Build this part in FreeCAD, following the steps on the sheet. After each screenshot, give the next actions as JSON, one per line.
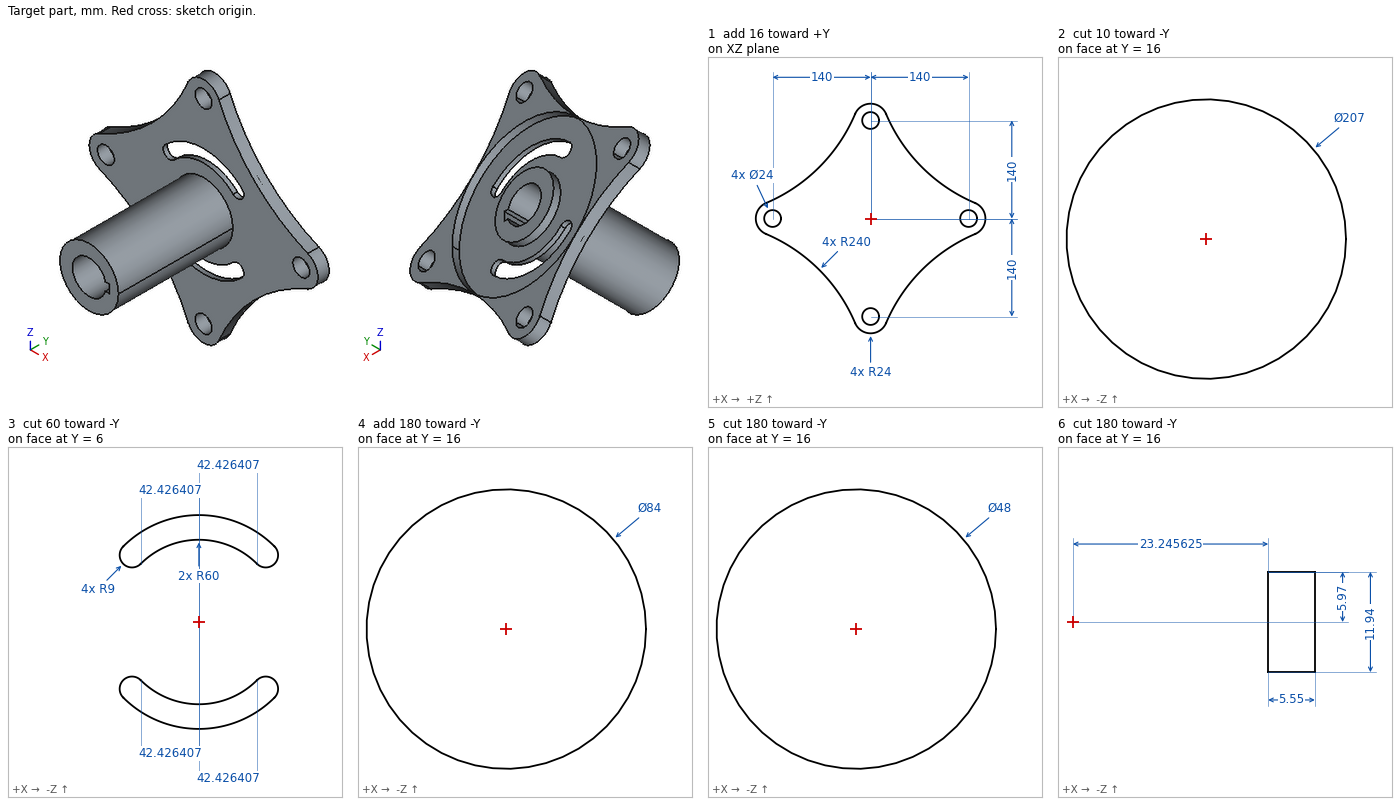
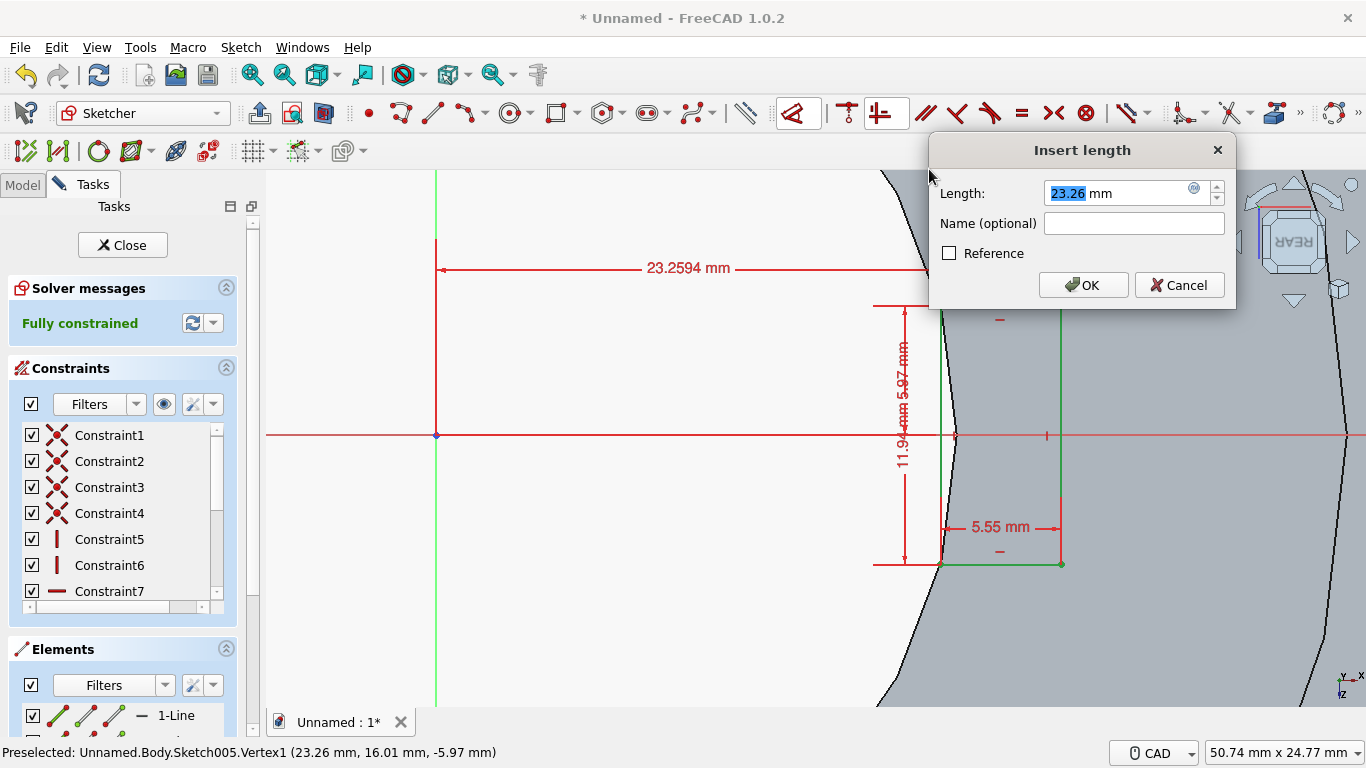
{"action": "type", "text": "23.245625"}
{"action": "key", "text": "Return"}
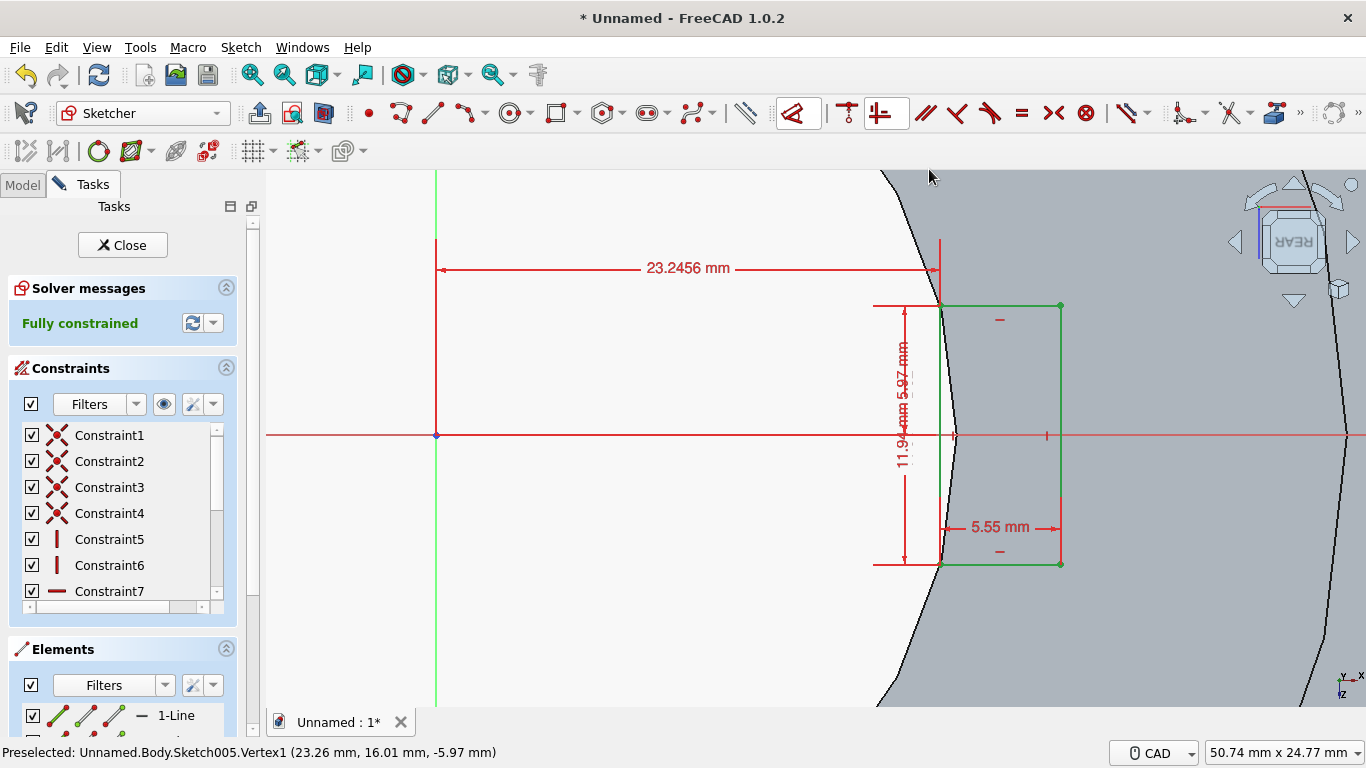
{"action": "left_click", "coordinate": [123, 245]}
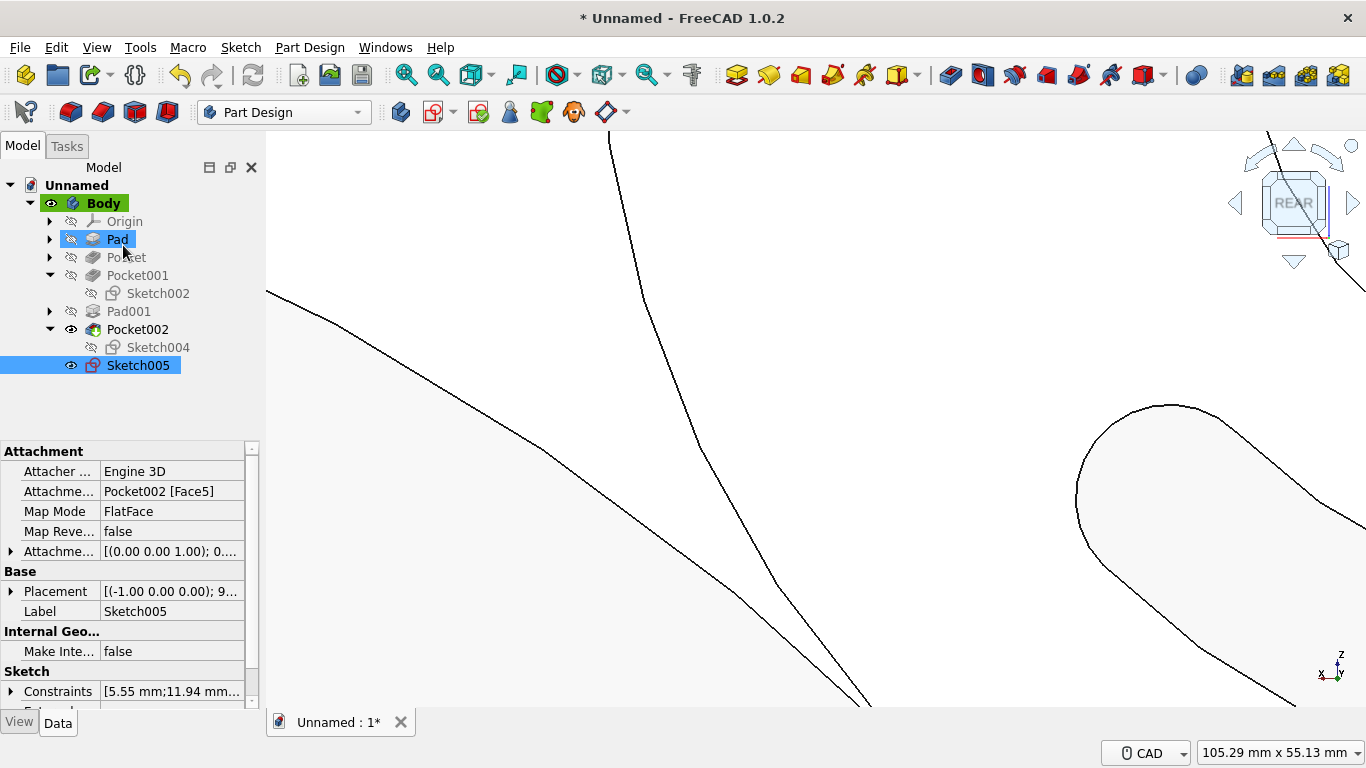
{"action": "left_click", "coordinate": [952, 76]}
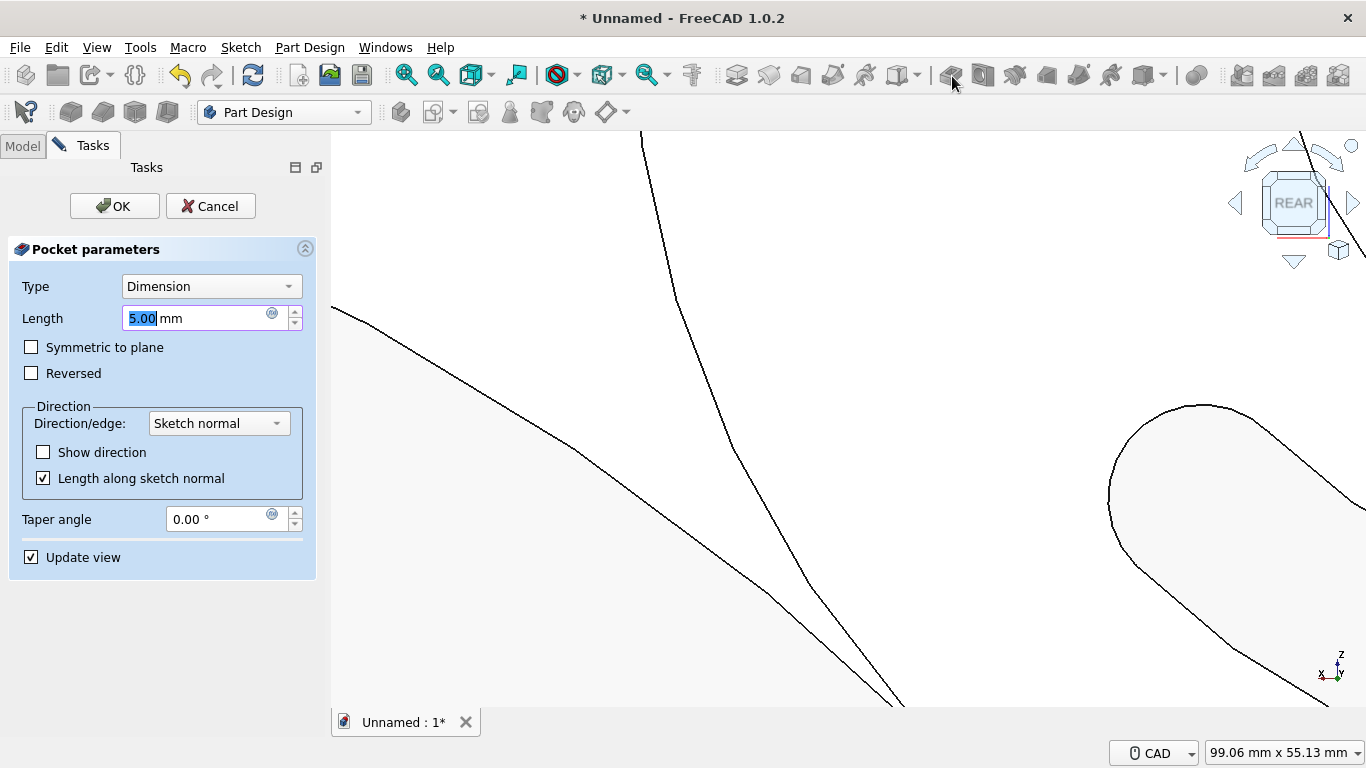
{"action": "type", "text": "180"}
{"action": "key", "text": "Tab"}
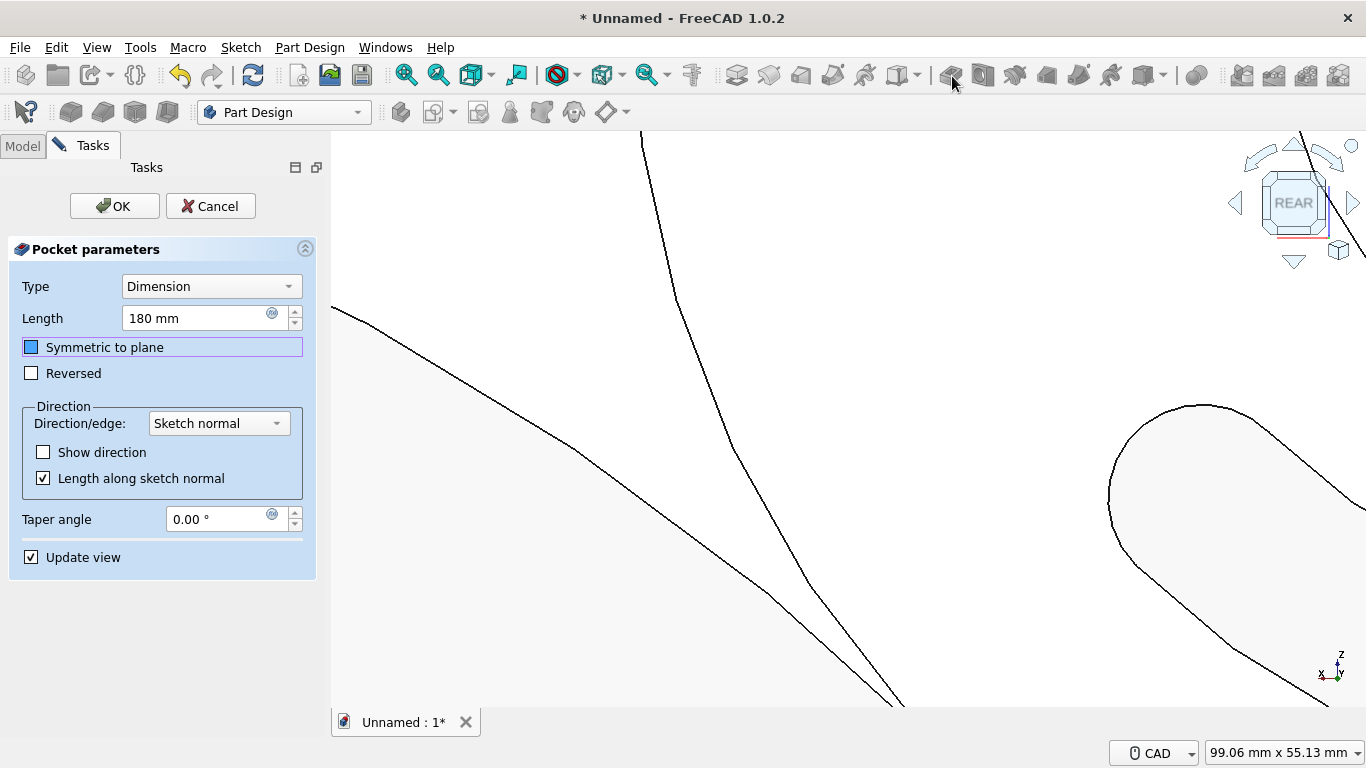
{"action": "left_click", "coordinate": [115, 206]}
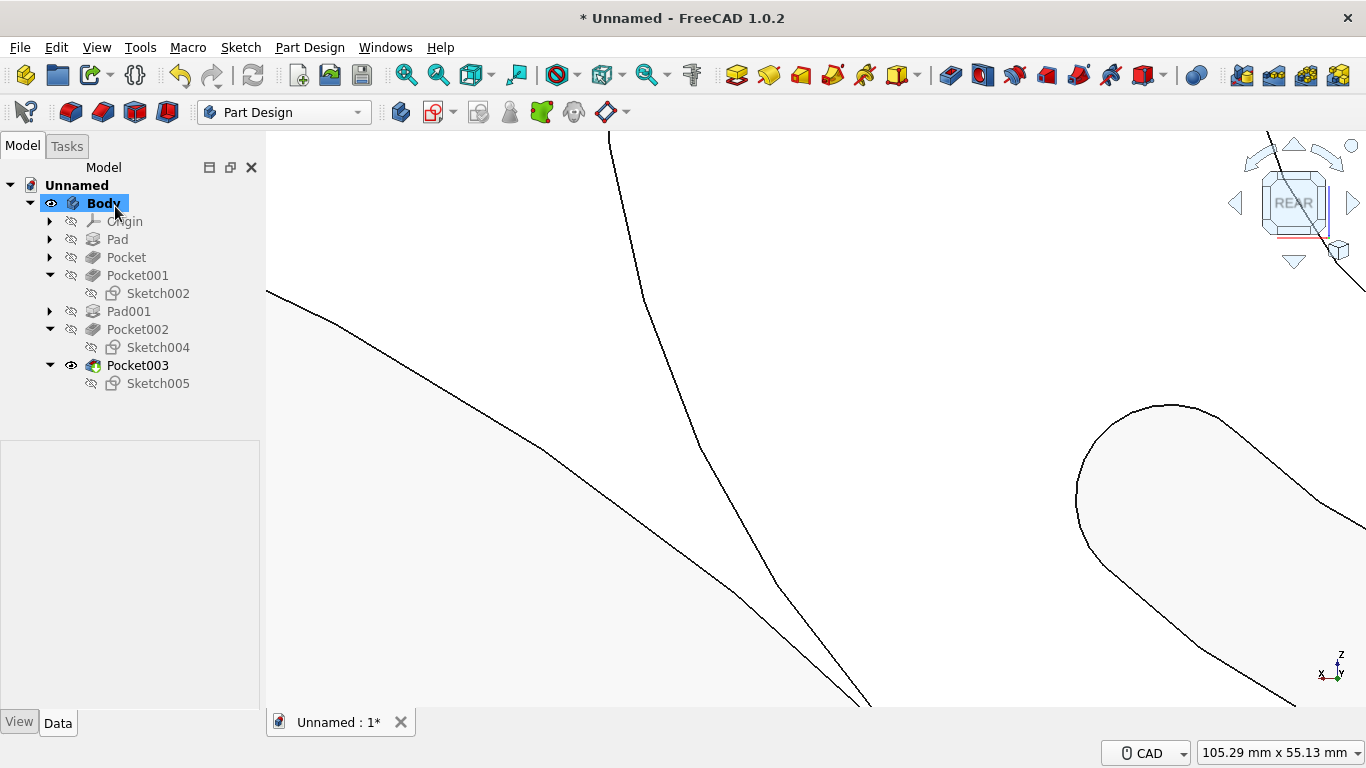
{"action": "key", "text": "0"}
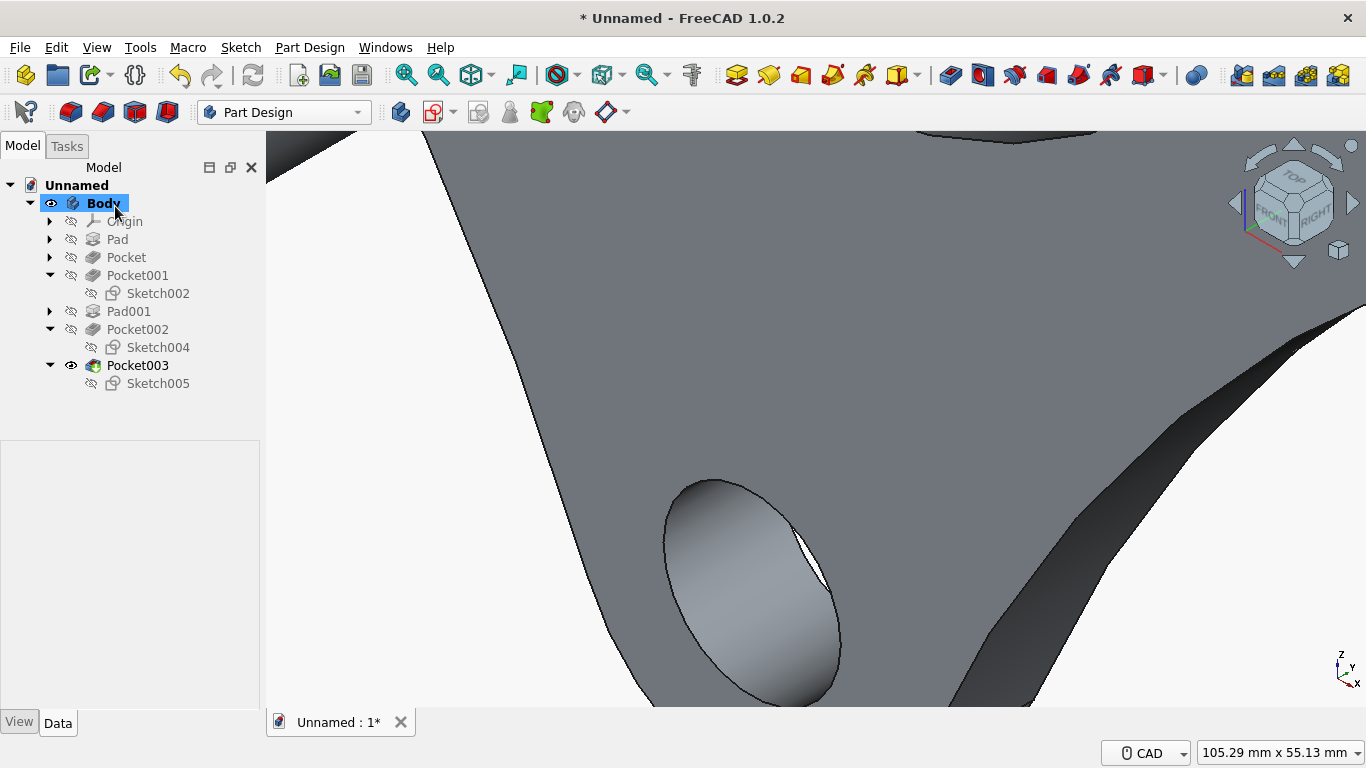
{"action": "left_click", "coordinate": [408, 76]}